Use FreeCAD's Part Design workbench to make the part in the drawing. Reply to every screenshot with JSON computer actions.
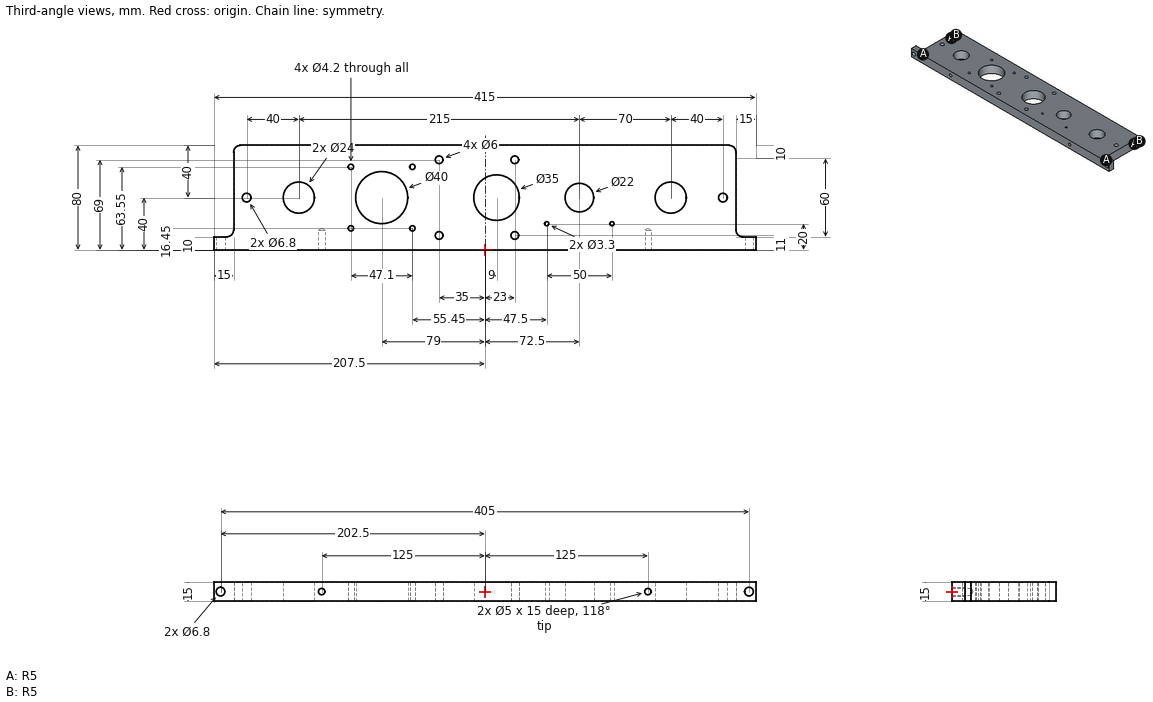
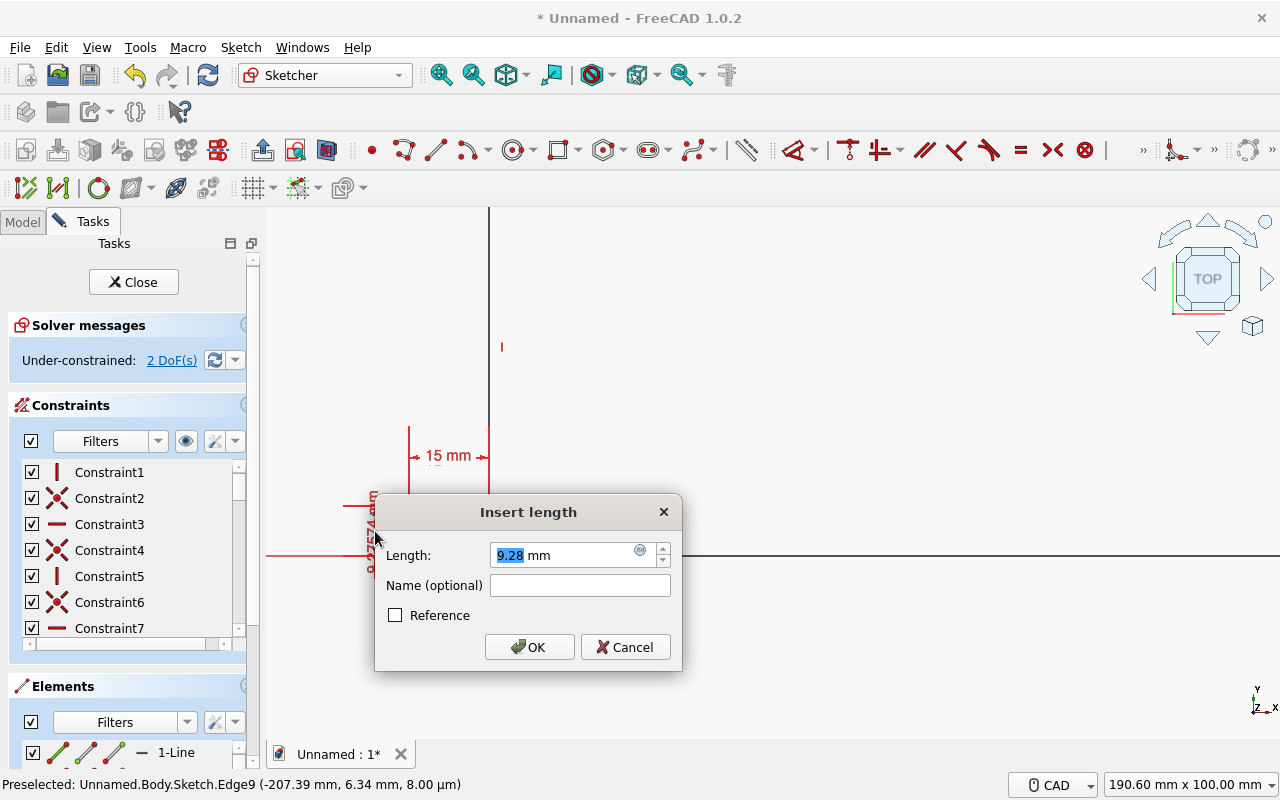
{"action": "type", "text": "10"}
{"action": "key", "text": "Return"}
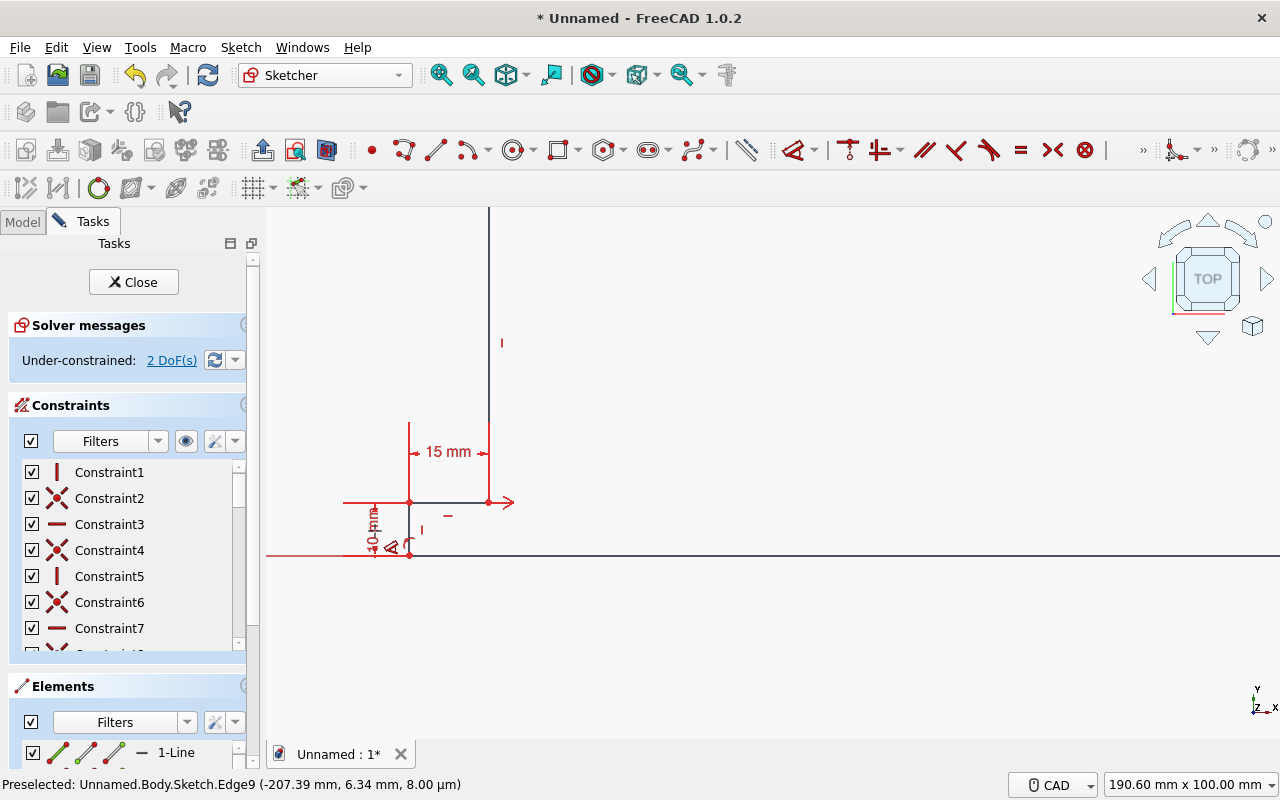
{"action": "scroll", "coordinate": [440, 516], "scroll_direction": "down", "scroll_amount": 7}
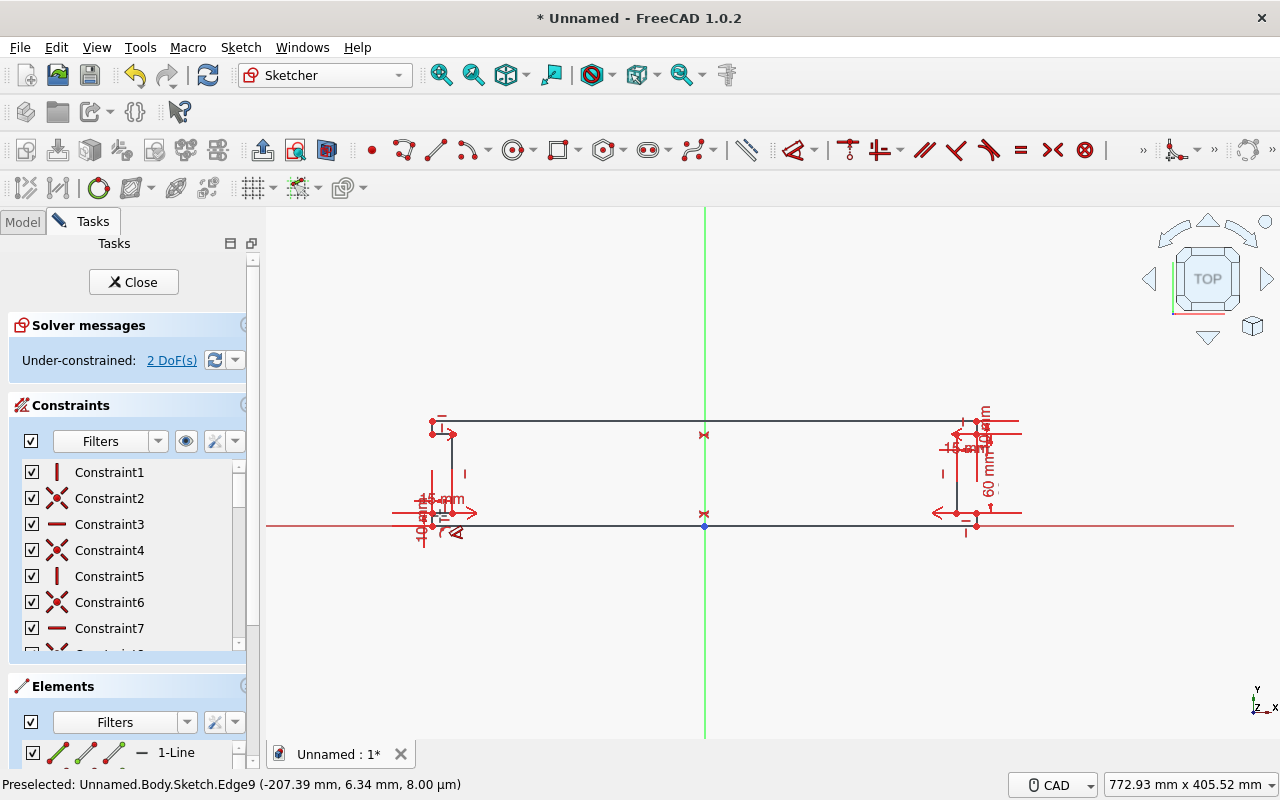
{"action": "scroll", "coordinate": [971, 513], "scroll_direction": "up", "scroll_amount": 5}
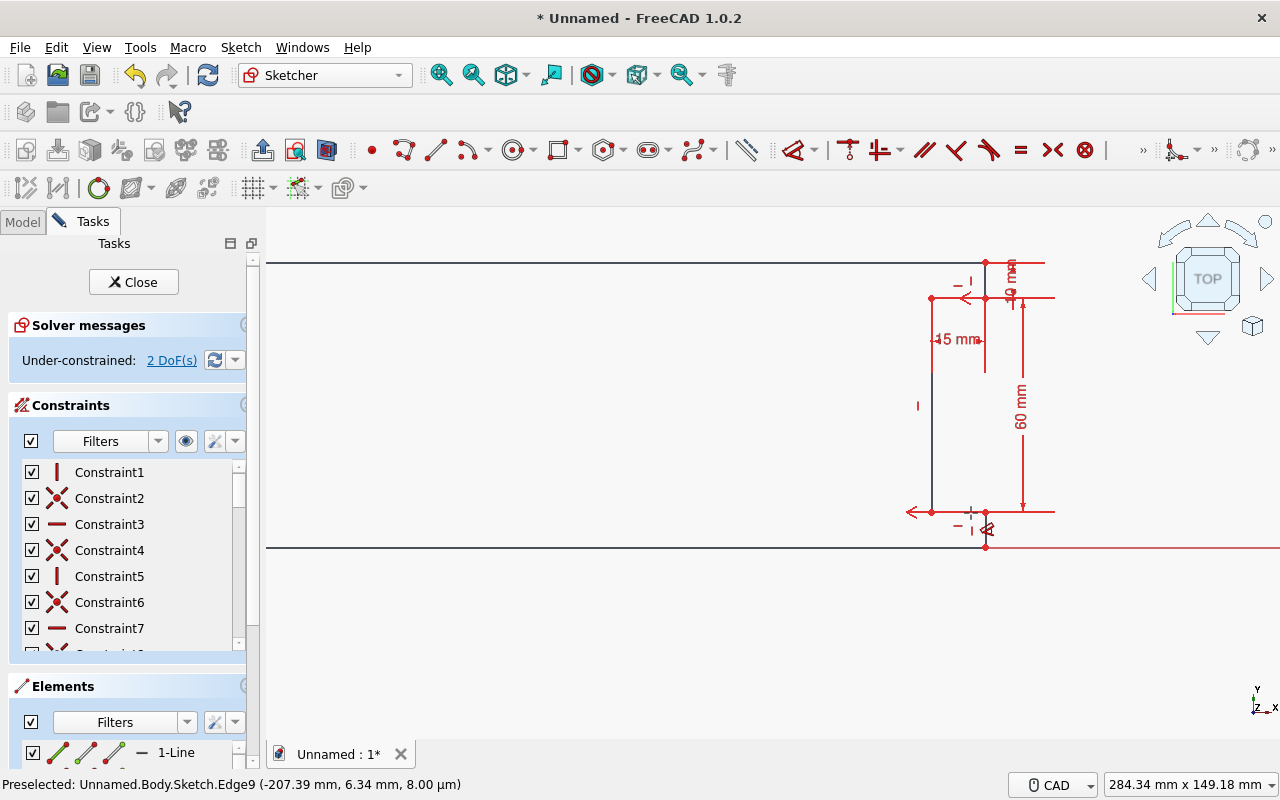
{"action": "left_click", "coordinate": [969, 512]}
{"action": "left_click", "coordinate": [959, 478]}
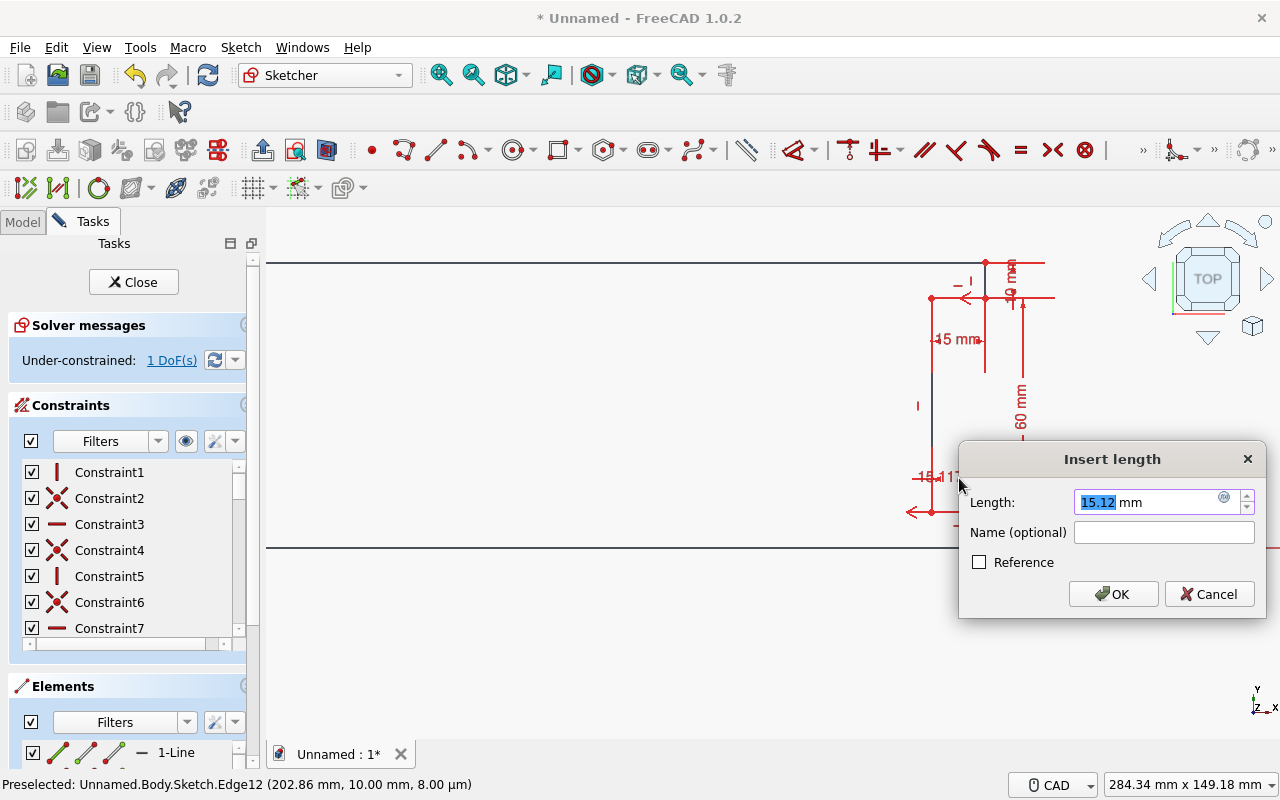
{"action": "type", "text": "15"}
{"action": "key", "text": "Return"}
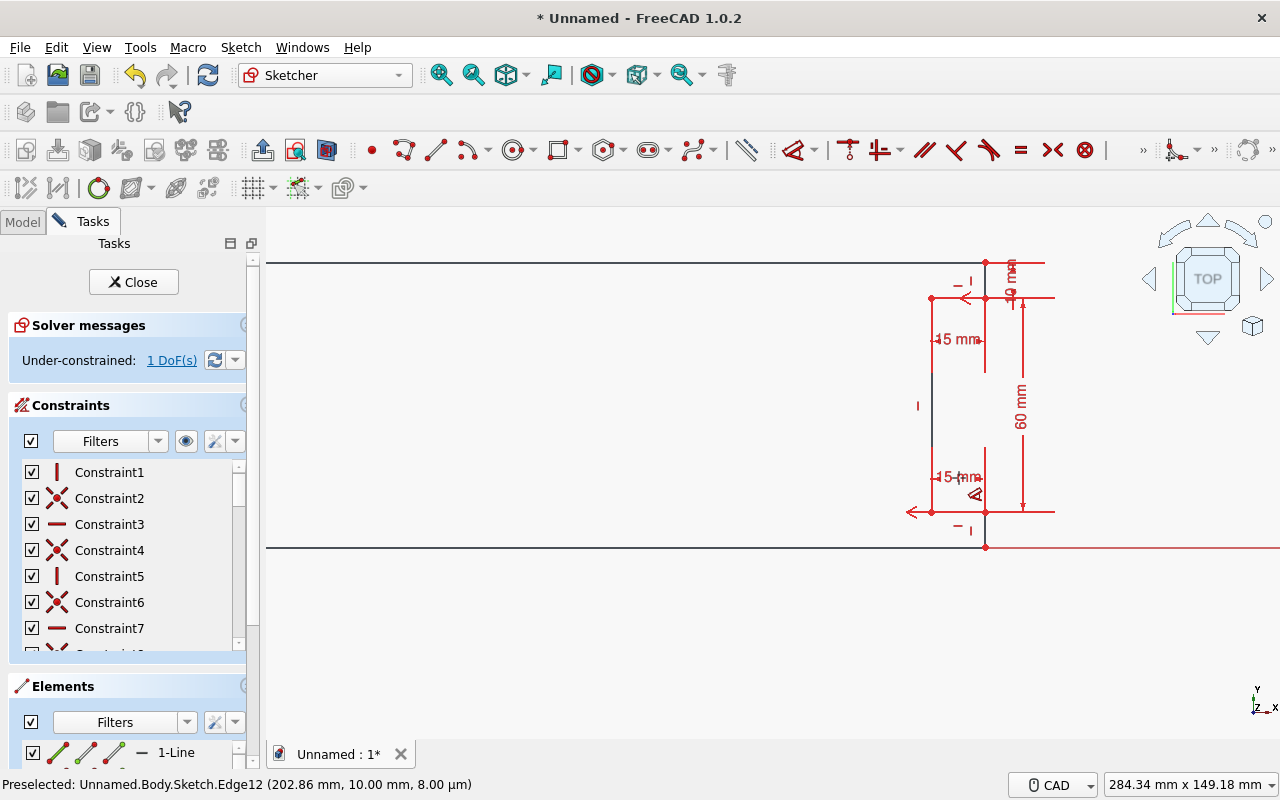
{"action": "left_click", "coordinate": [541, 263]}
{"action": "left_click", "coordinate": [640, 297]}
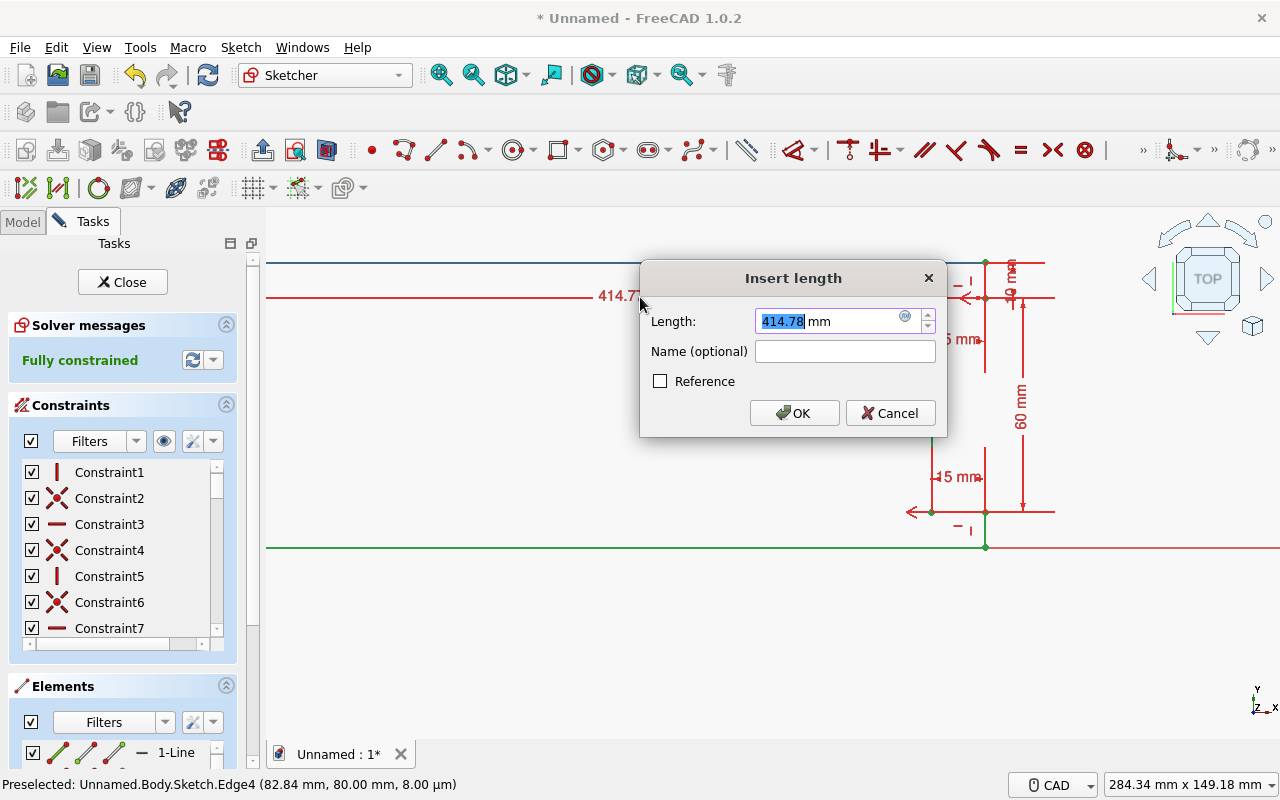
{"action": "type", "text": "415"}
{"action": "key", "text": "Return"}
{"action": "key", "text": "Escape"}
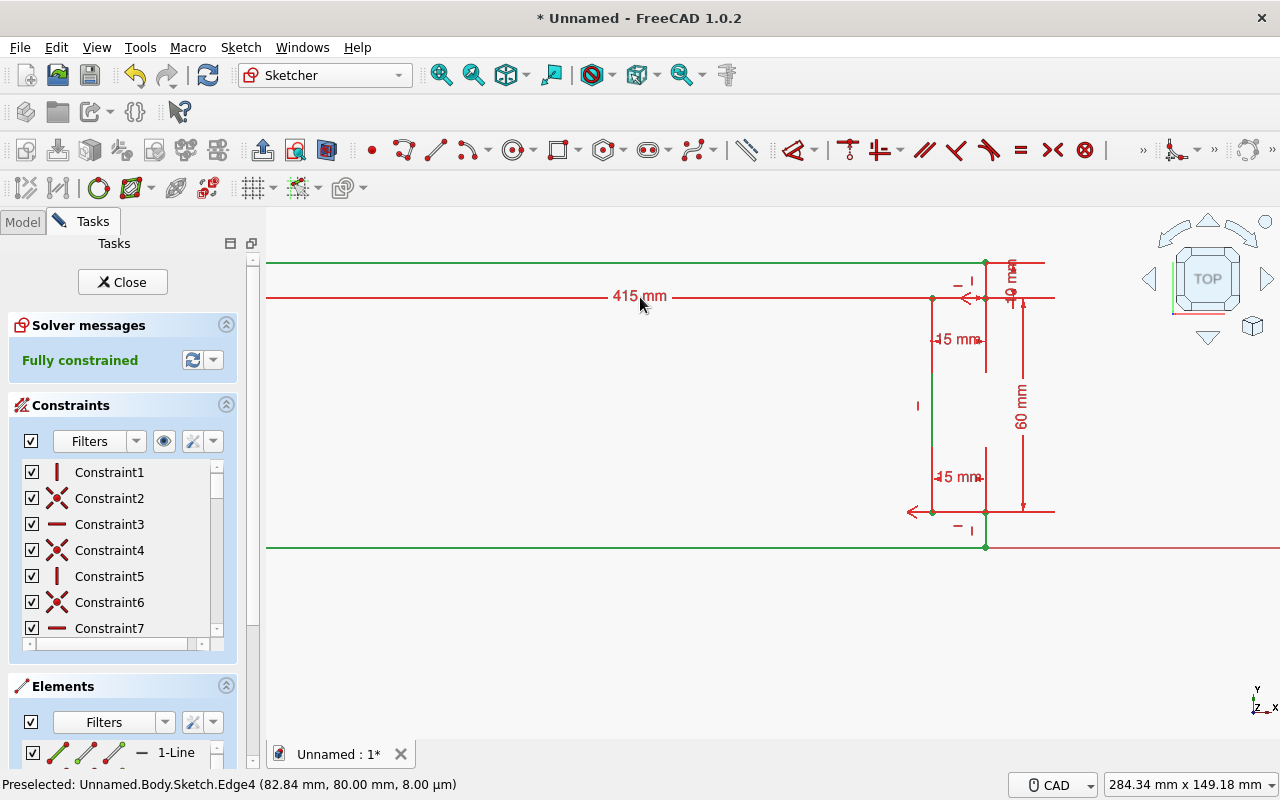
{"action": "left_click", "coordinate": [123, 282]}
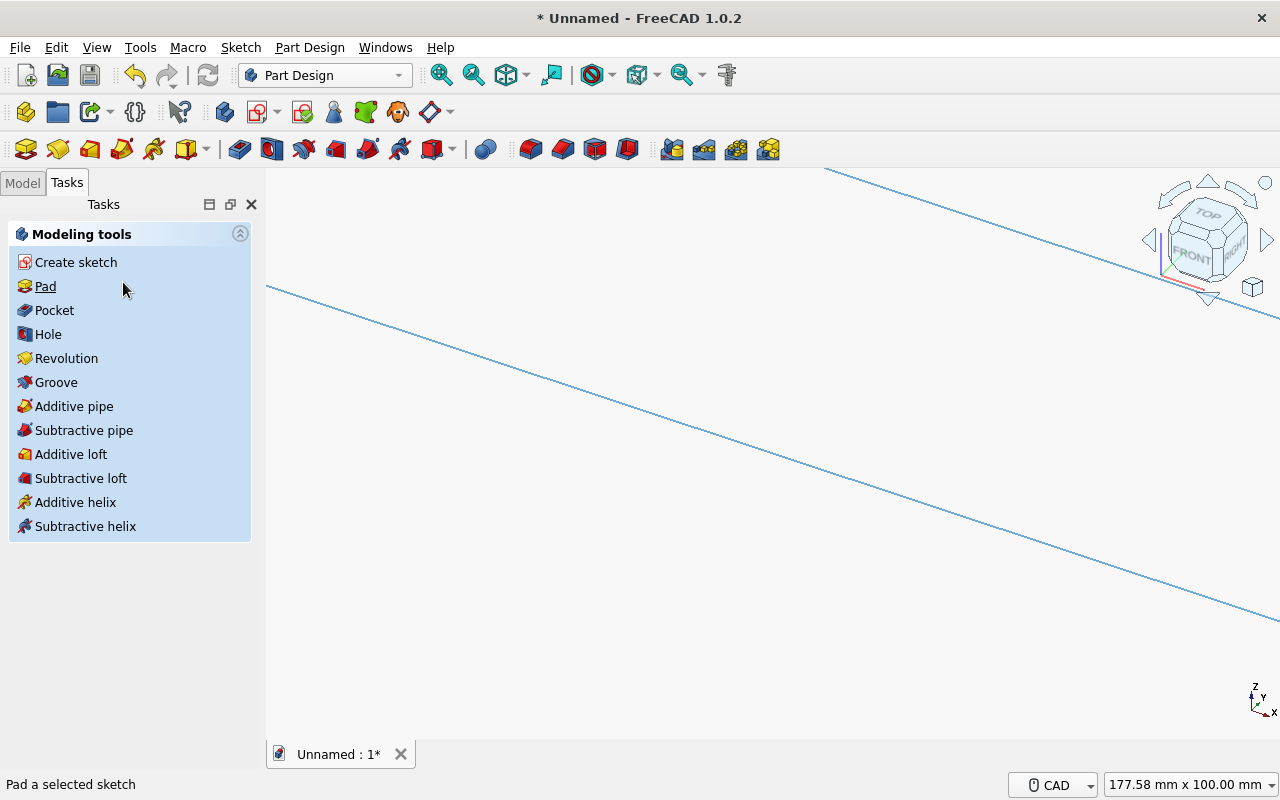
{"action": "left_click", "coordinate": [26, 150]}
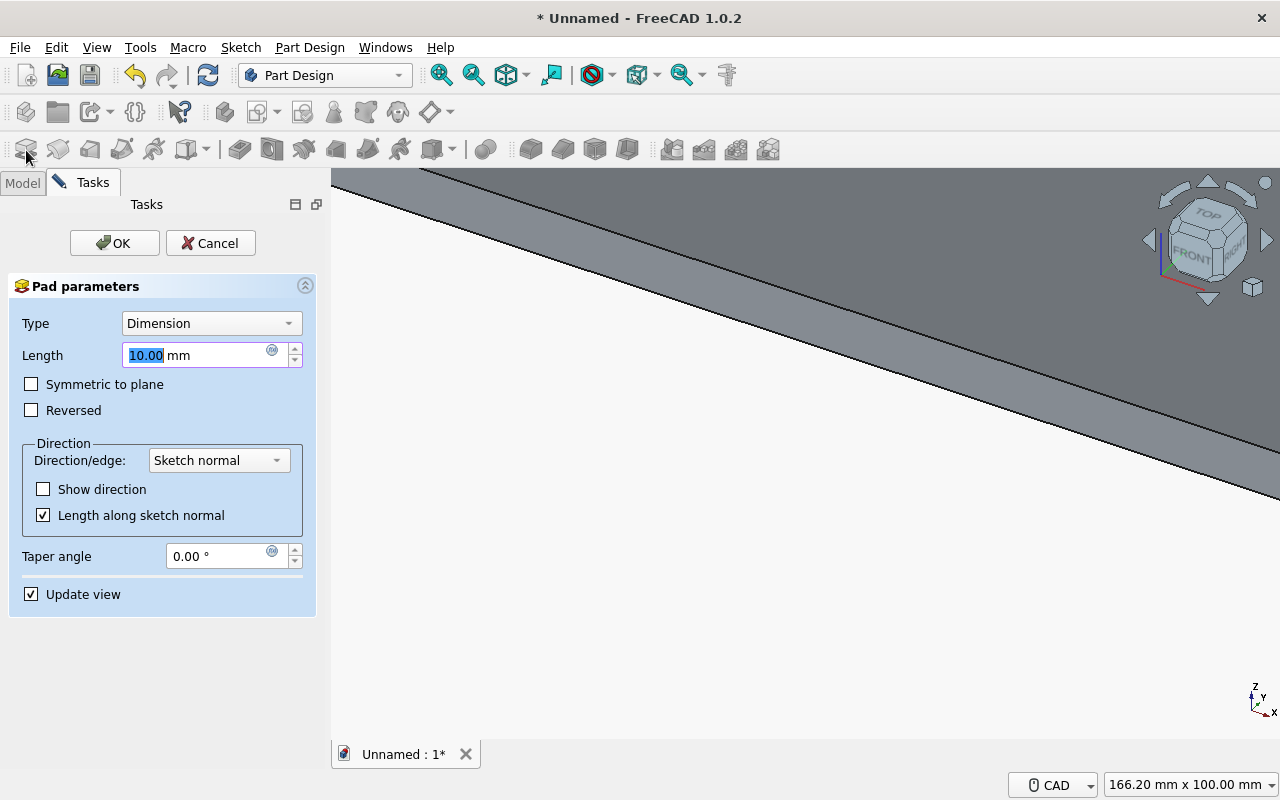
{"action": "type", "text": "15"}
{"action": "key", "text": "Tab"}